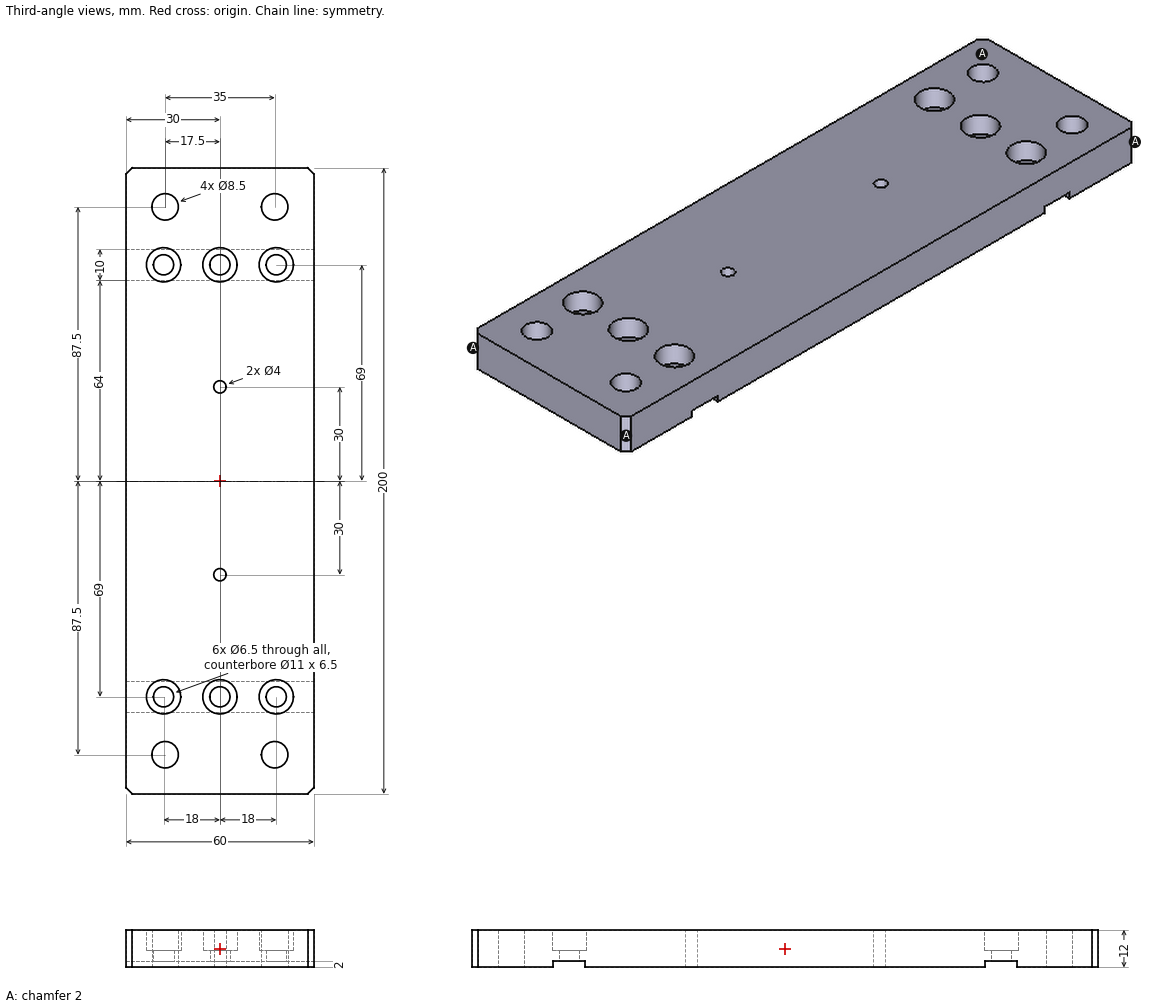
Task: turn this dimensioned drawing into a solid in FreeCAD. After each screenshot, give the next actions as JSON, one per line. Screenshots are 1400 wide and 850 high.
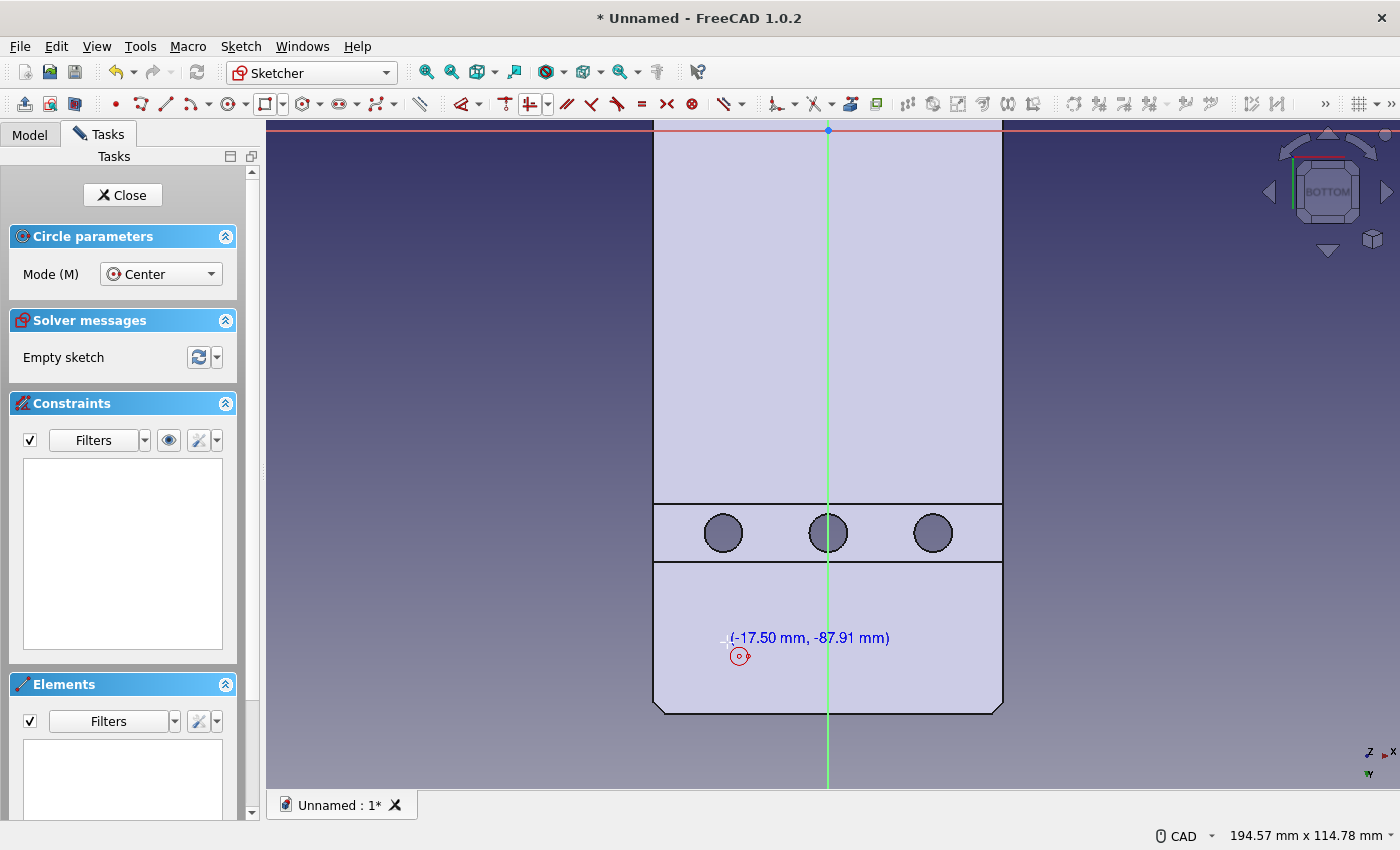
{"action": "left_click", "coordinate": [726, 641]}
{"action": "left_click", "coordinate": [744, 623]}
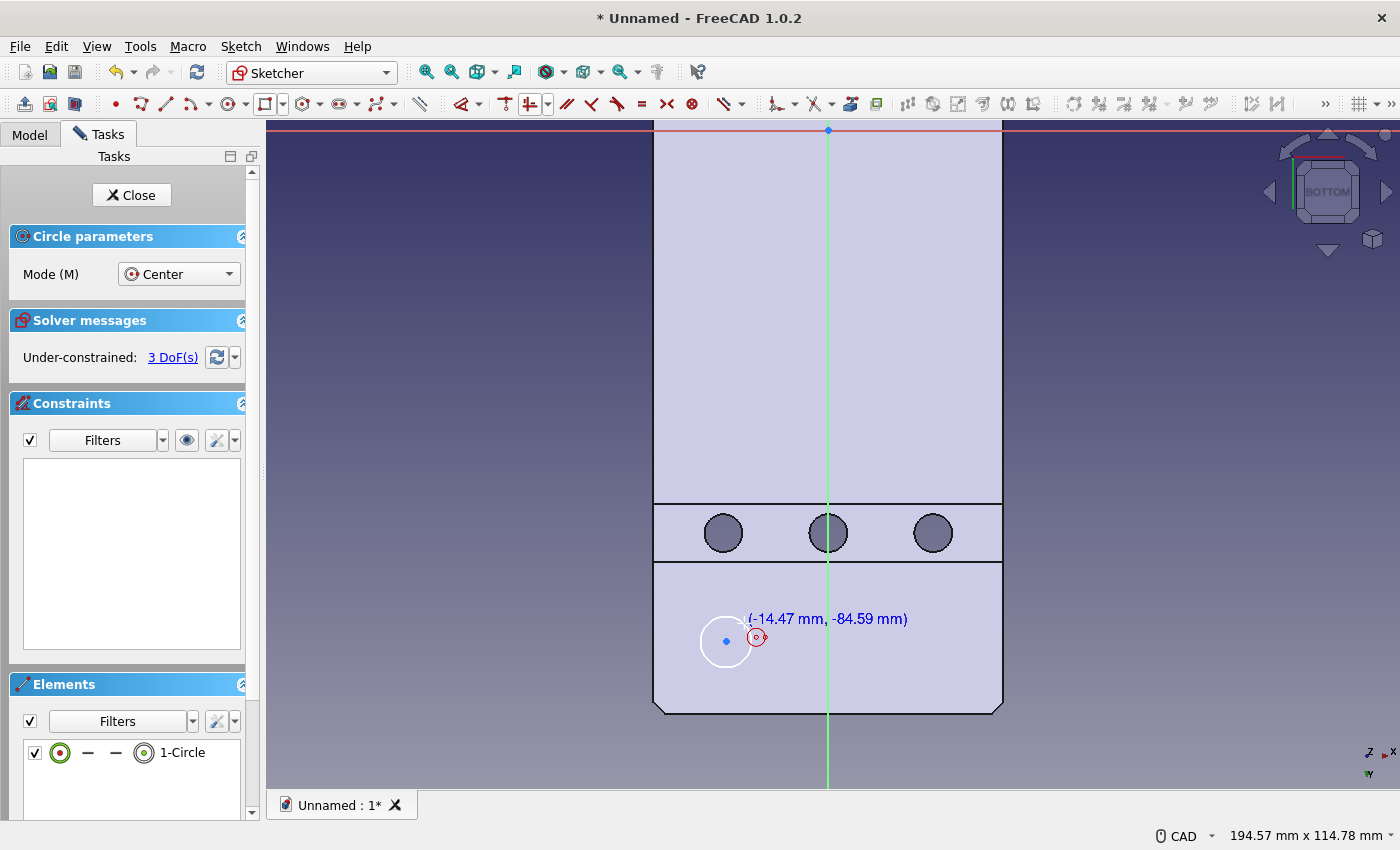
{"action": "left_click", "coordinate": [930, 641]}
{"action": "left_click", "coordinate": [948, 623]}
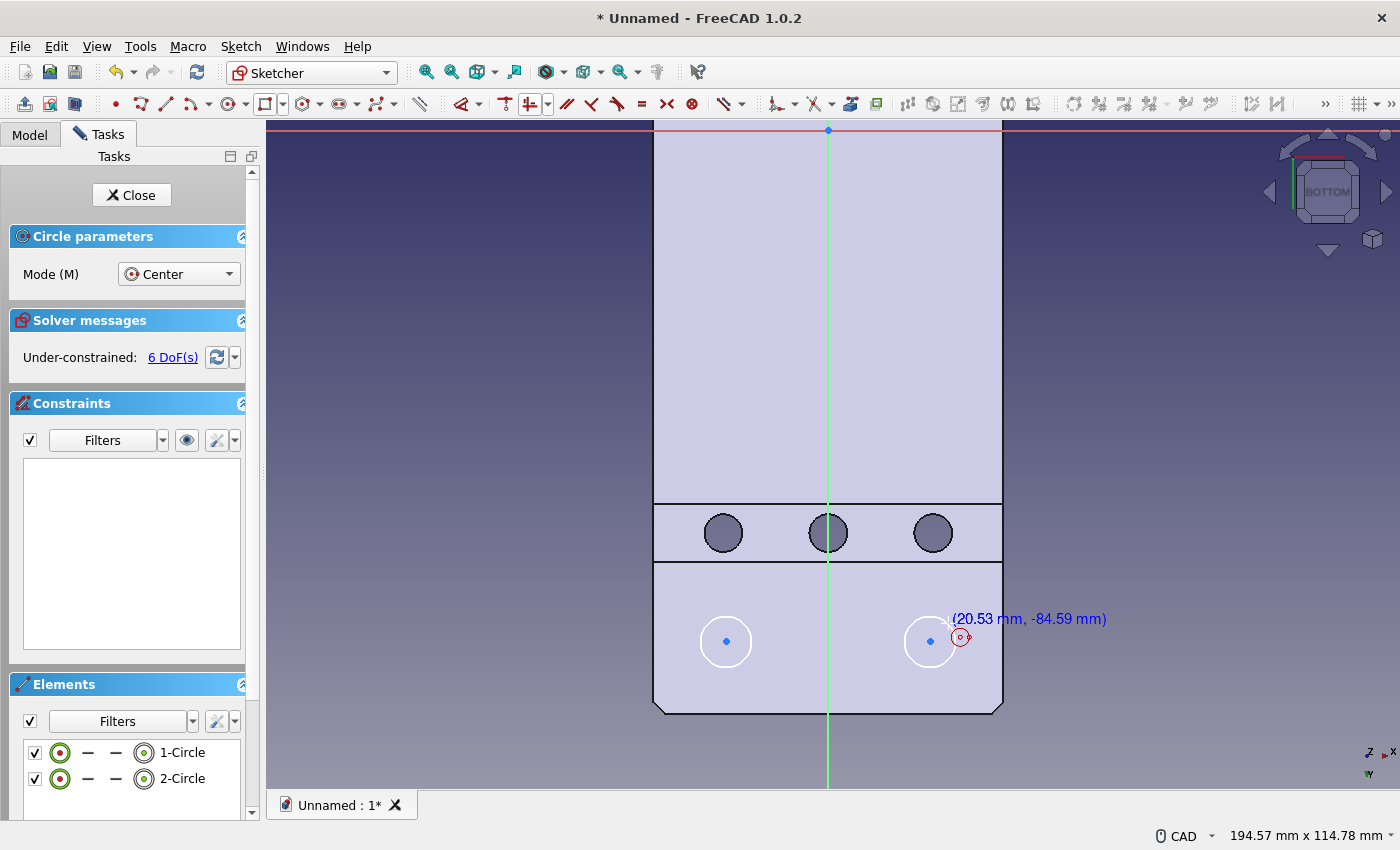
{"action": "scroll", "coordinate": [727, 643], "scroll_direction": "down", "scroll_amount": 5}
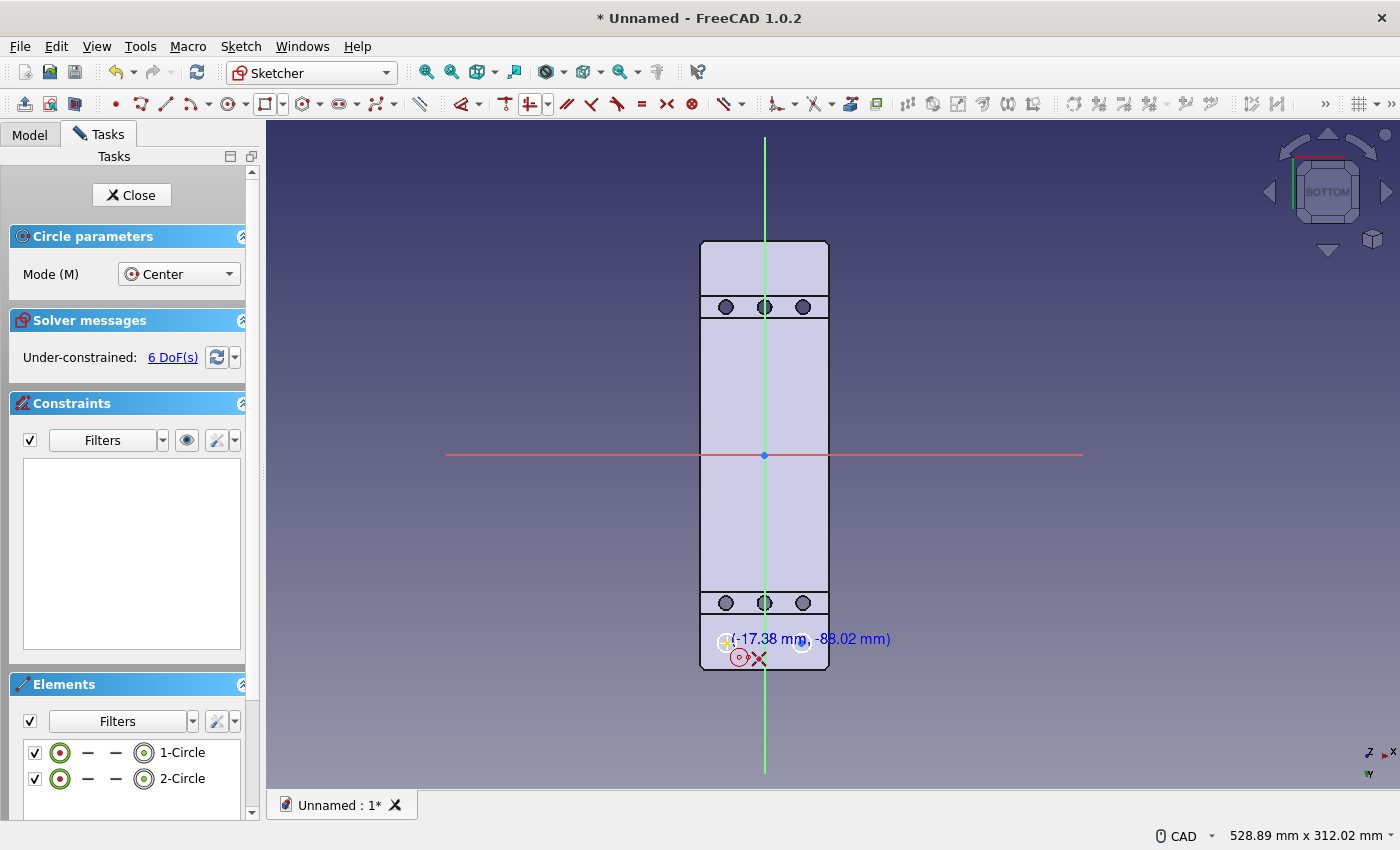
{"action": "scroll", "coordinate": [727, 268], "scroll_direction": "up", "scroll_amount": 5}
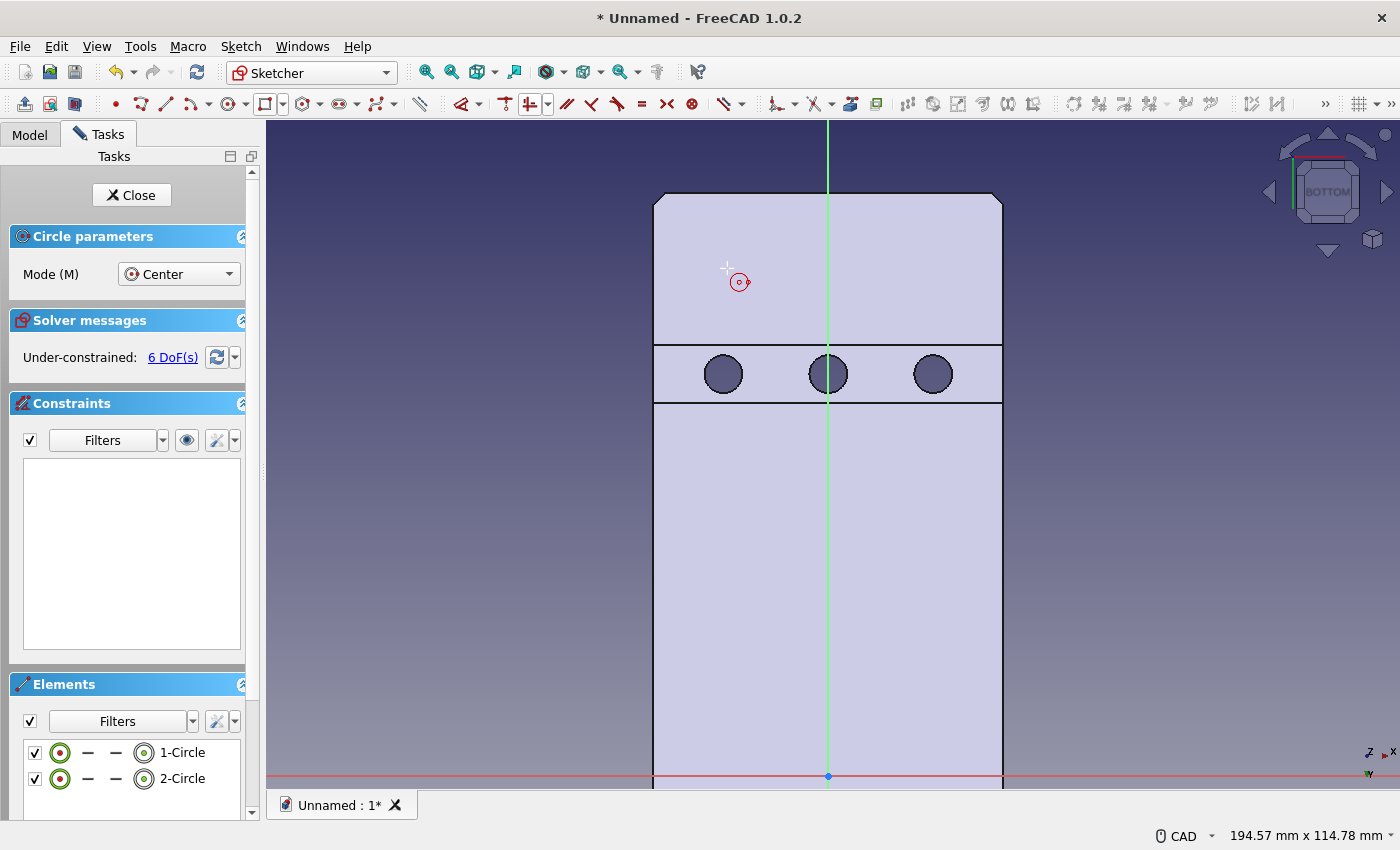
{"action": "left_click", "coordinate": [726, 266]}
{"action": "left_click", "coordinate": [744, 249]}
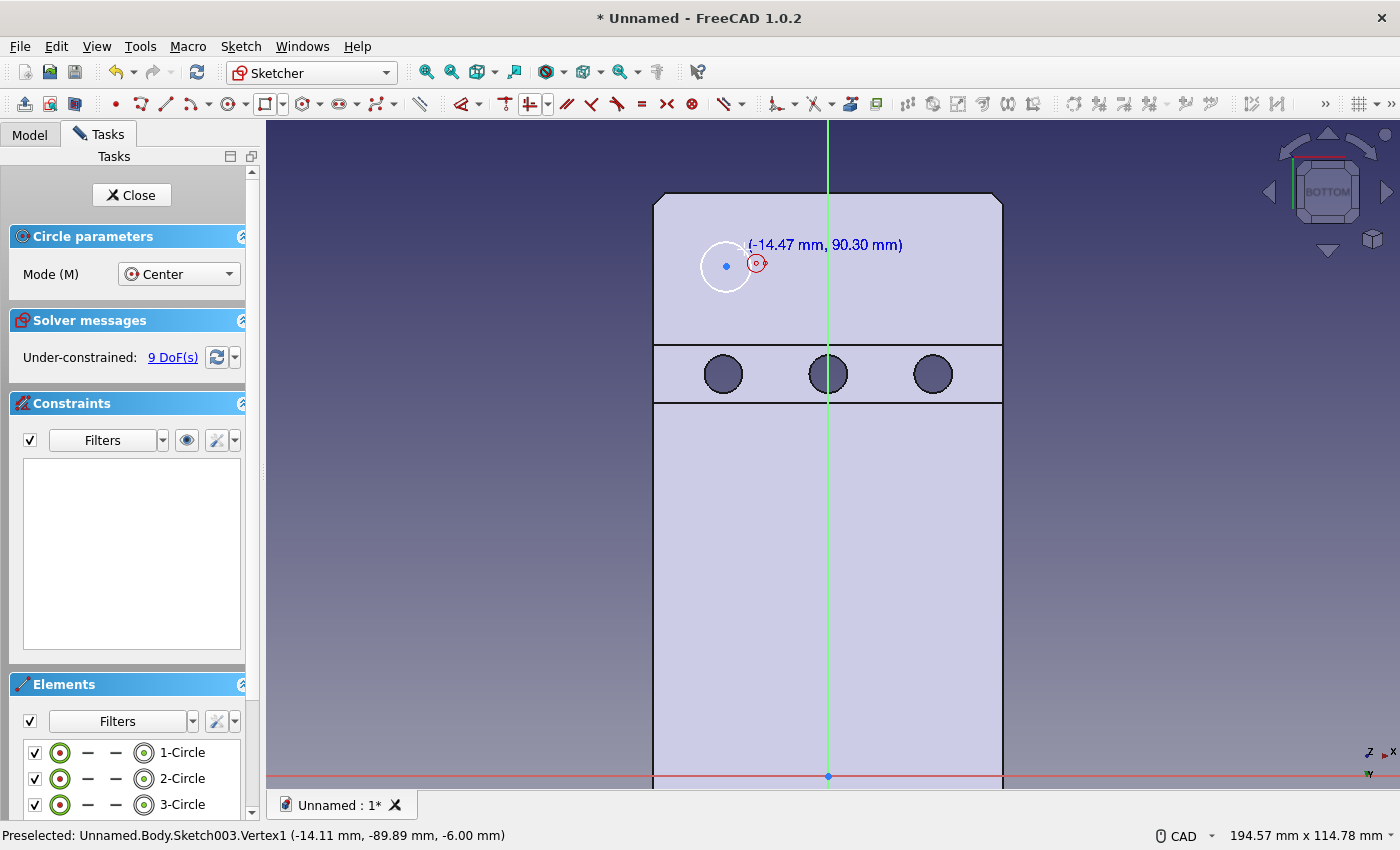
{"action": "left_click", "coordinate": [930, 266]}
{"action": "left_click", "coordinate": [948, 249]}
{"action": "key", "text": "Escape"}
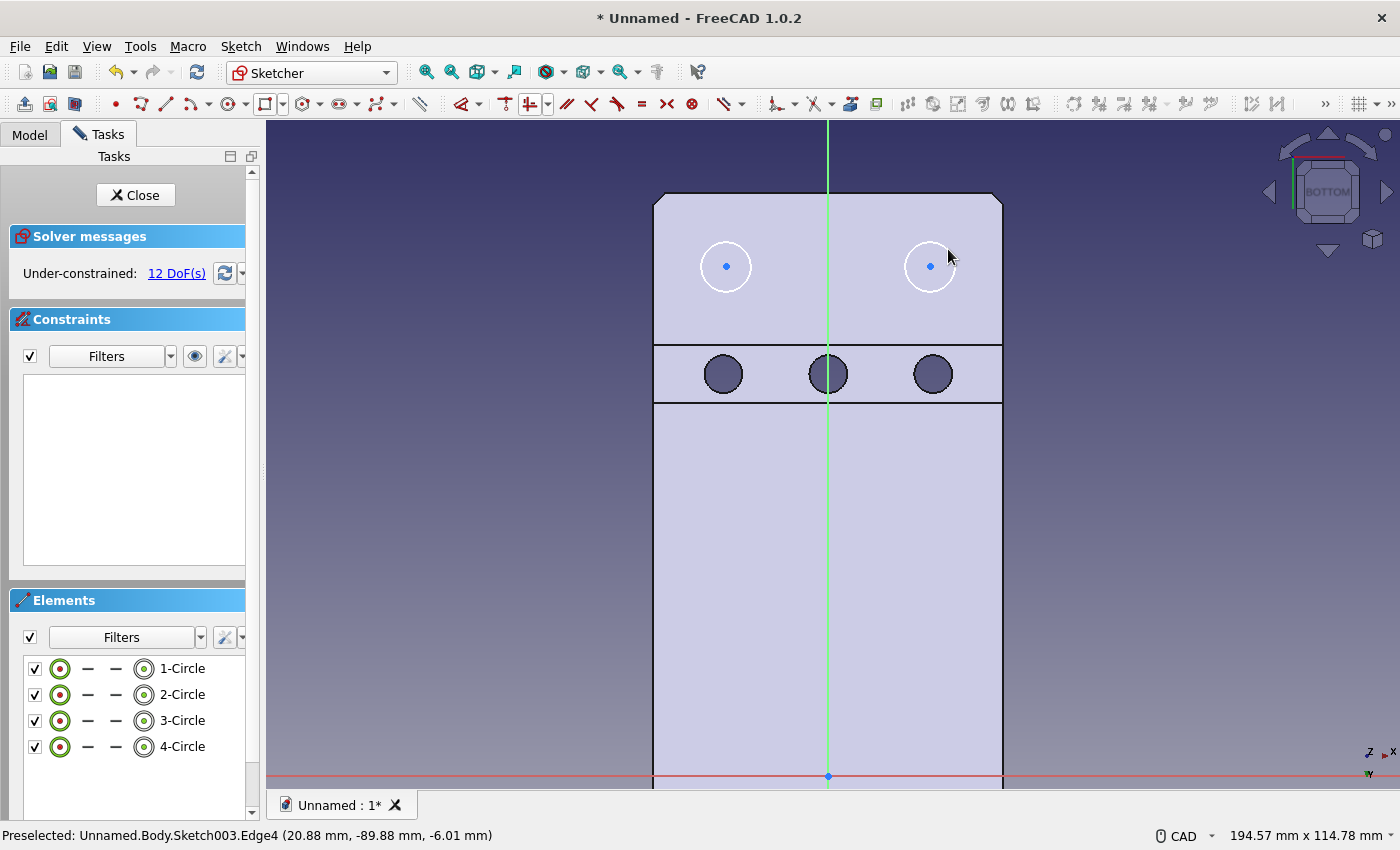
{"action": "scroll", "coordinate": [727, 267], "scroll_direction": "down", "scroll_amount": 5}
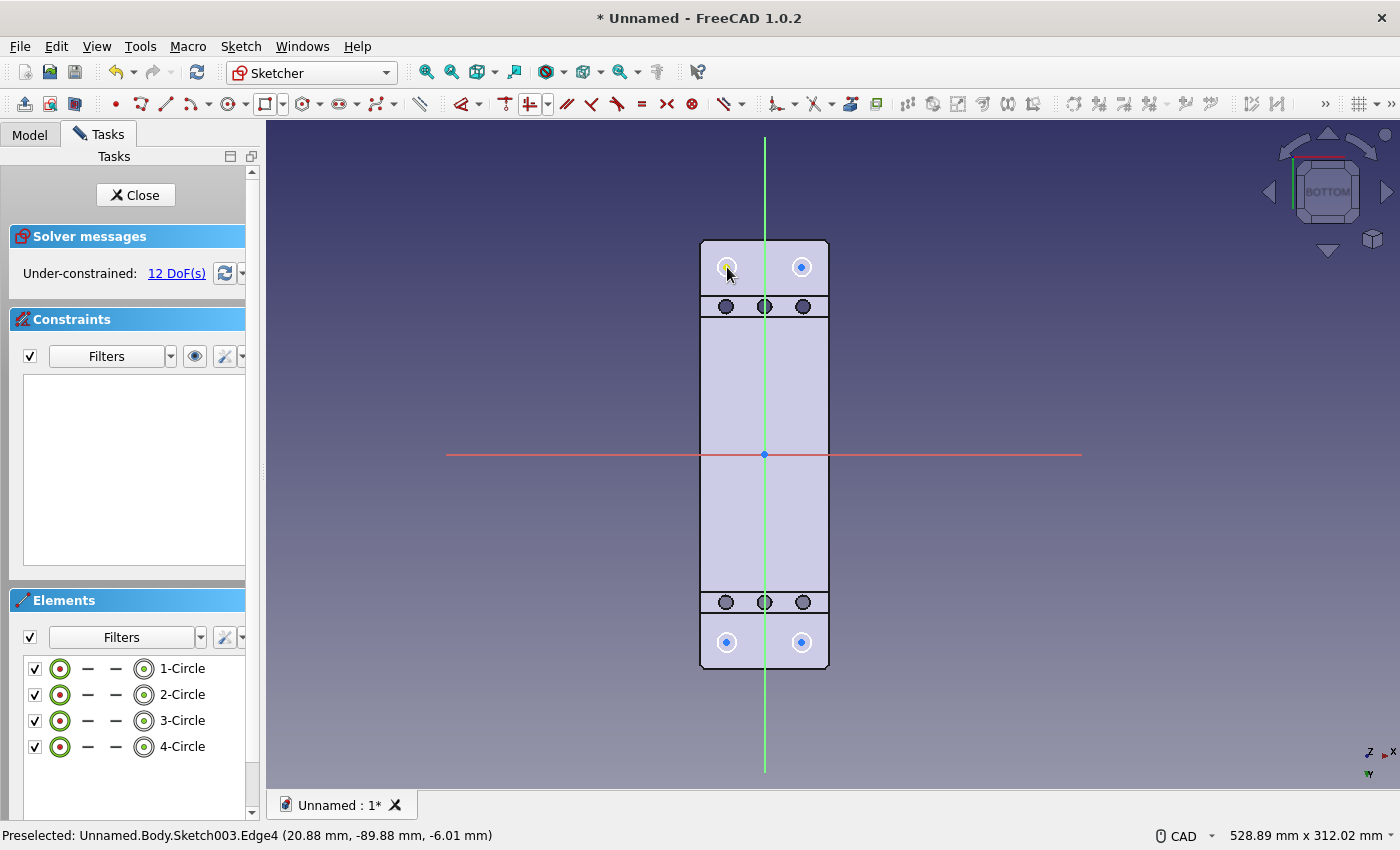
{"action": "scroll", "coordinate": [733, 636], "scroll_direction": "up", "scroll_amount": 2}